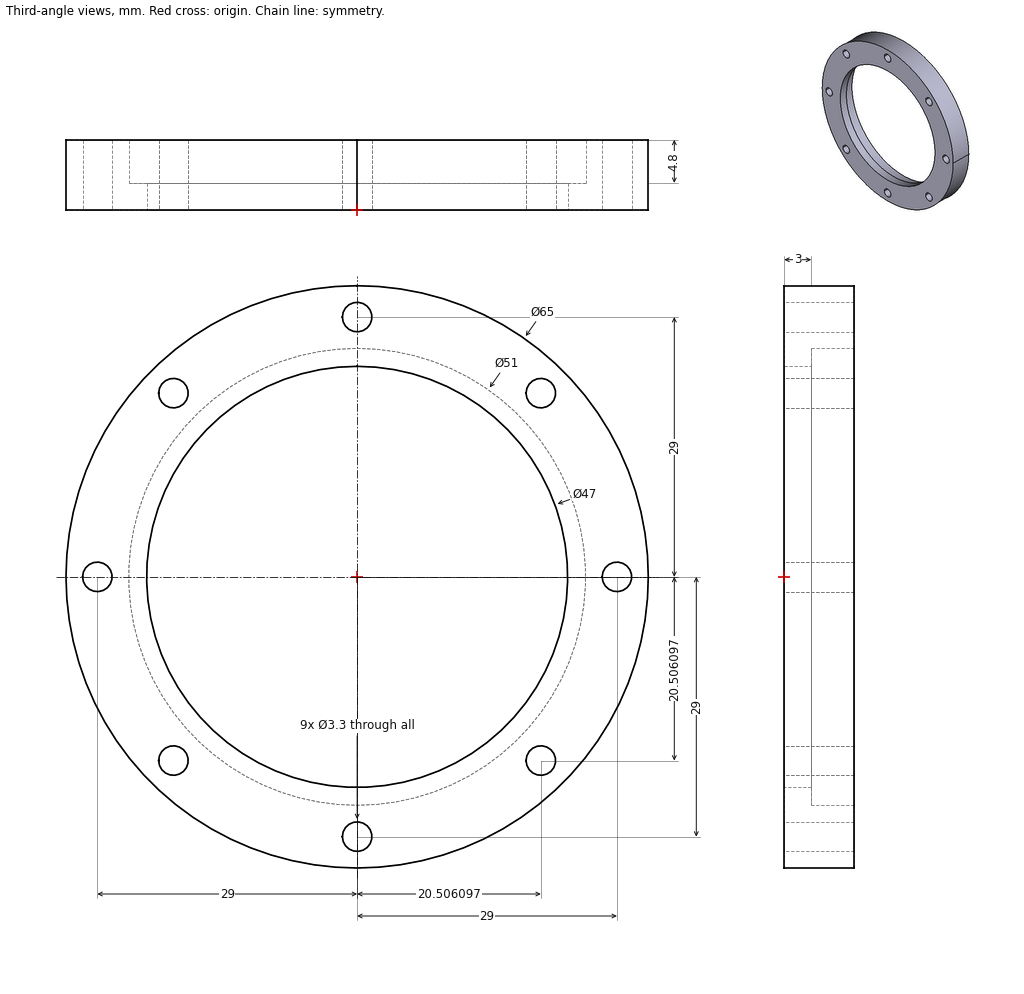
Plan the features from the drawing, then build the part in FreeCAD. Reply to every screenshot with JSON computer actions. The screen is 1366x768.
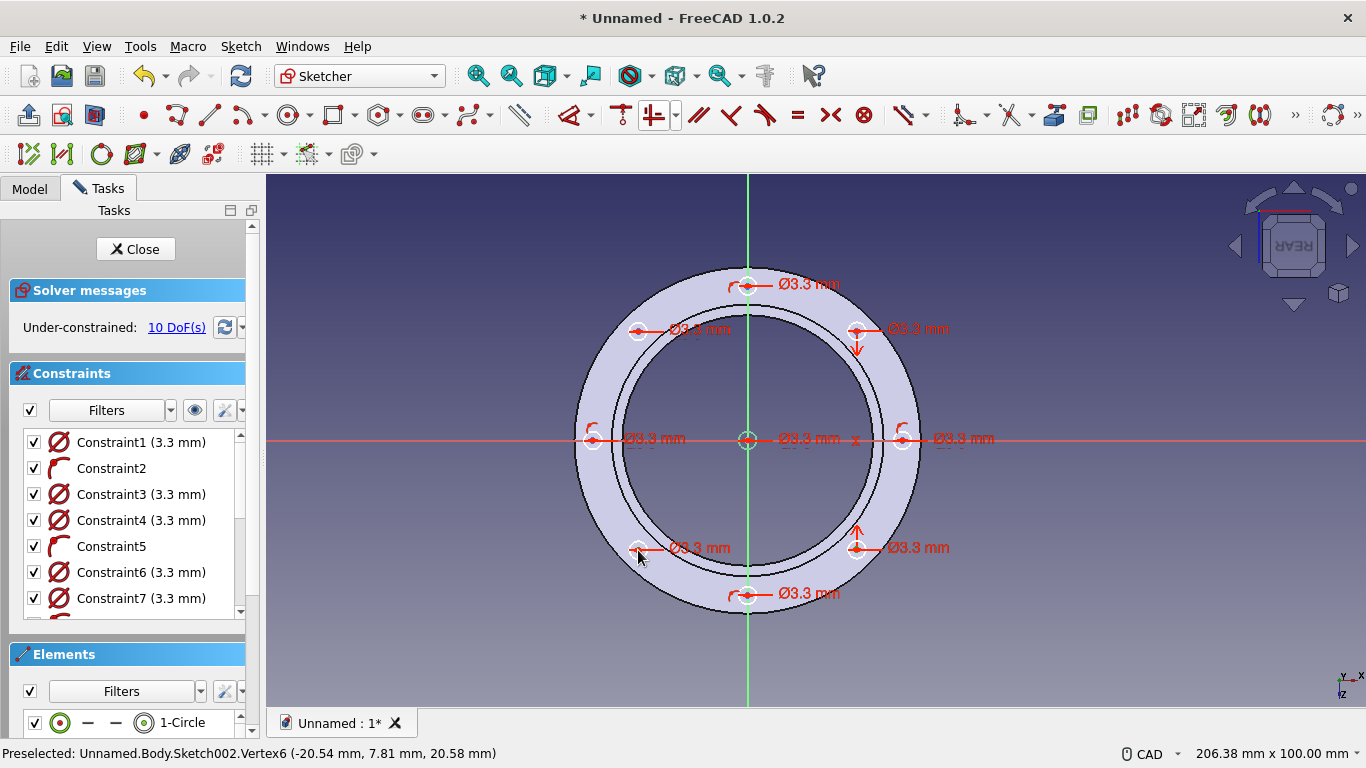
{"action": "left_click", "coordinate": [748, 645]}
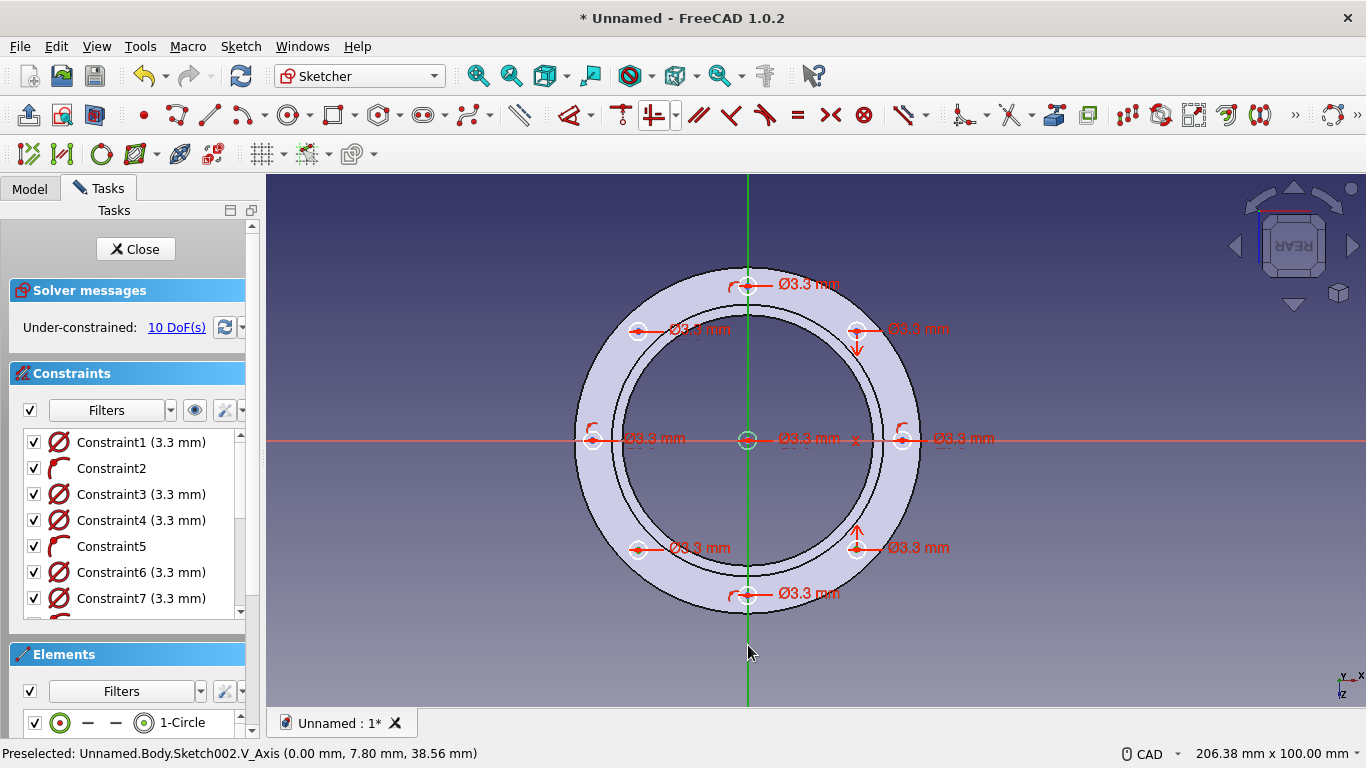
{"action": "left_click", "coordinate": [831, 116]}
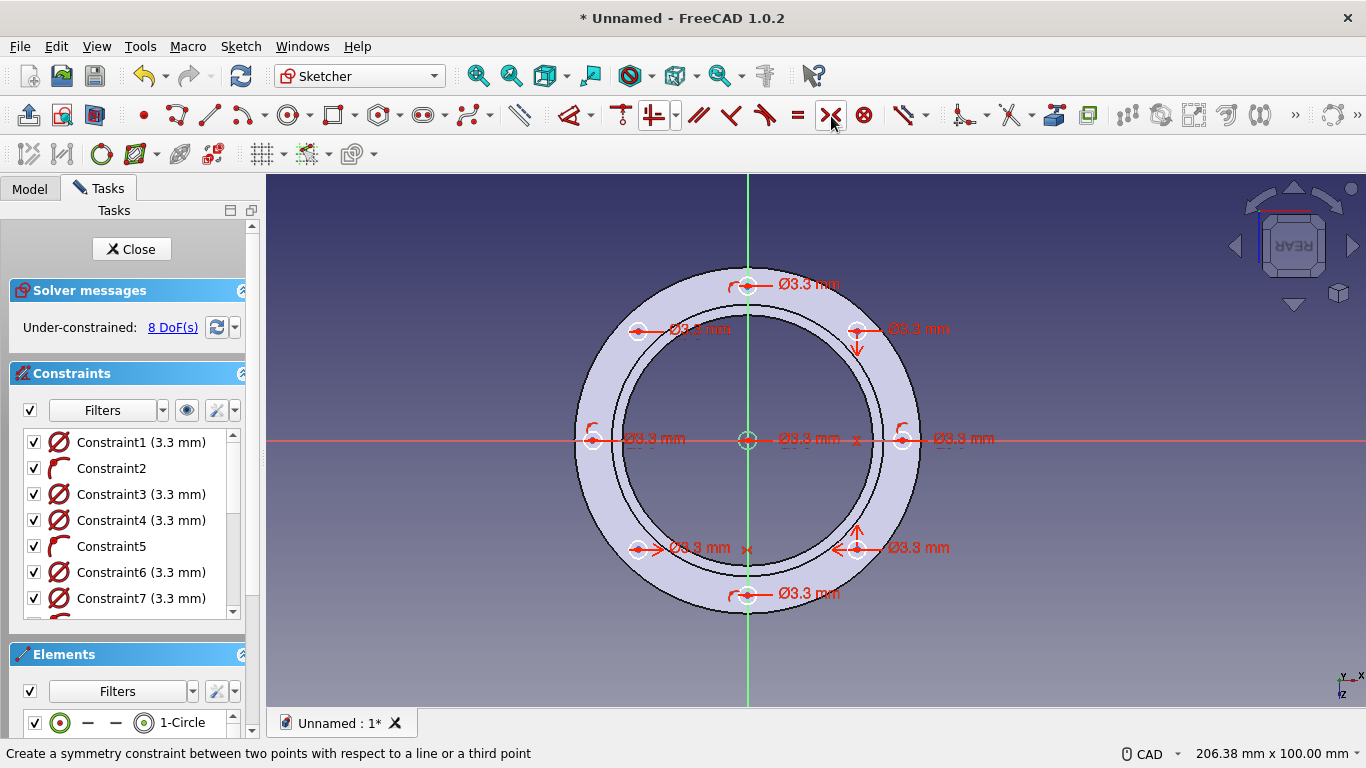
{"action": "left_click", "coordinate": [857, 331]}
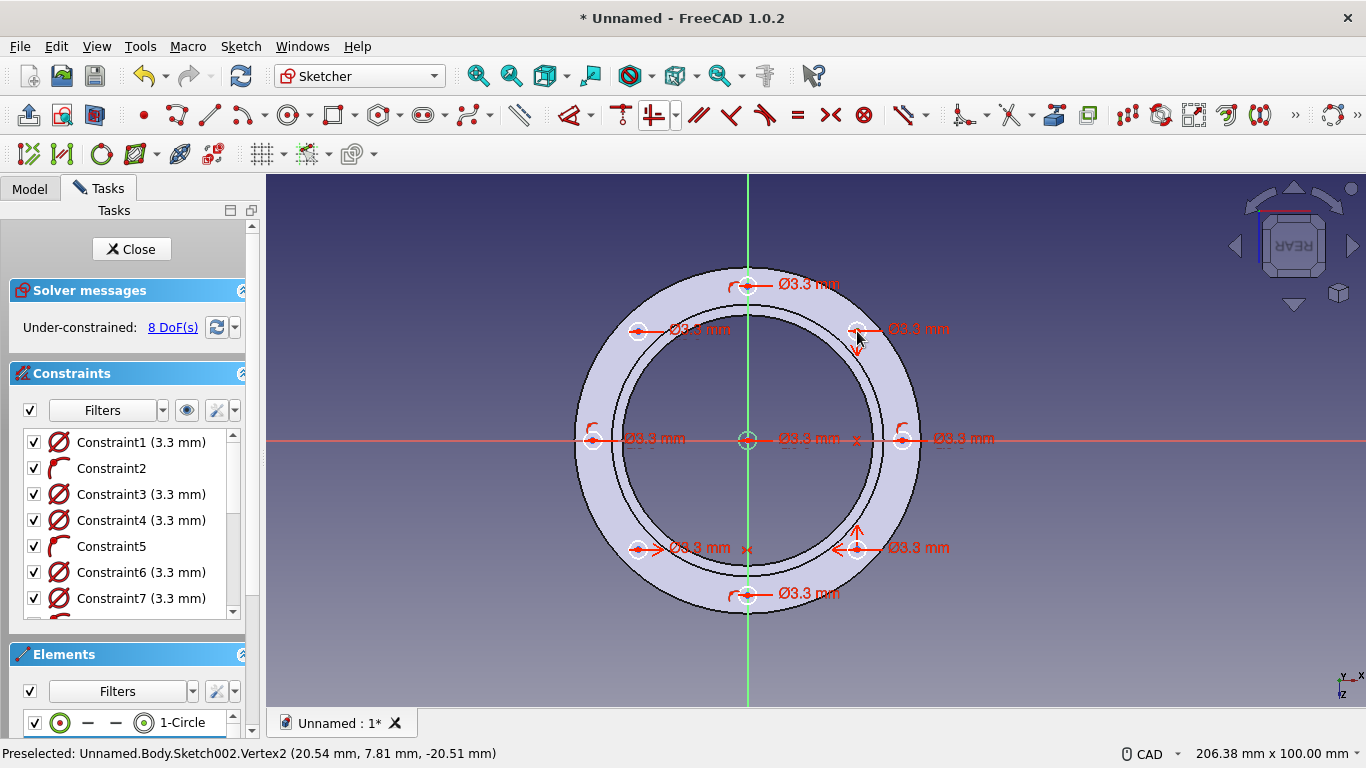
{"action": "left_click", "coordinate": [638, 332]}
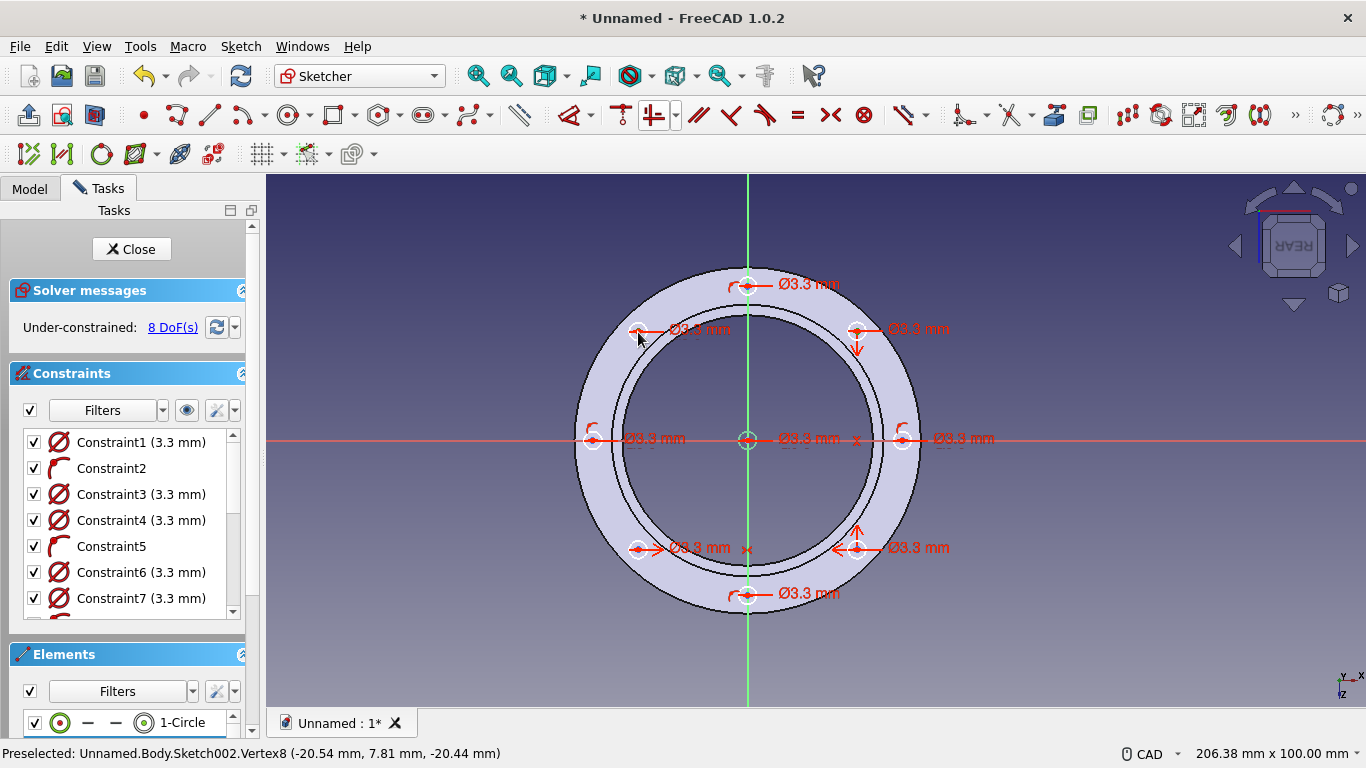
{"action": "left_click", "coordinate": [748, 645]}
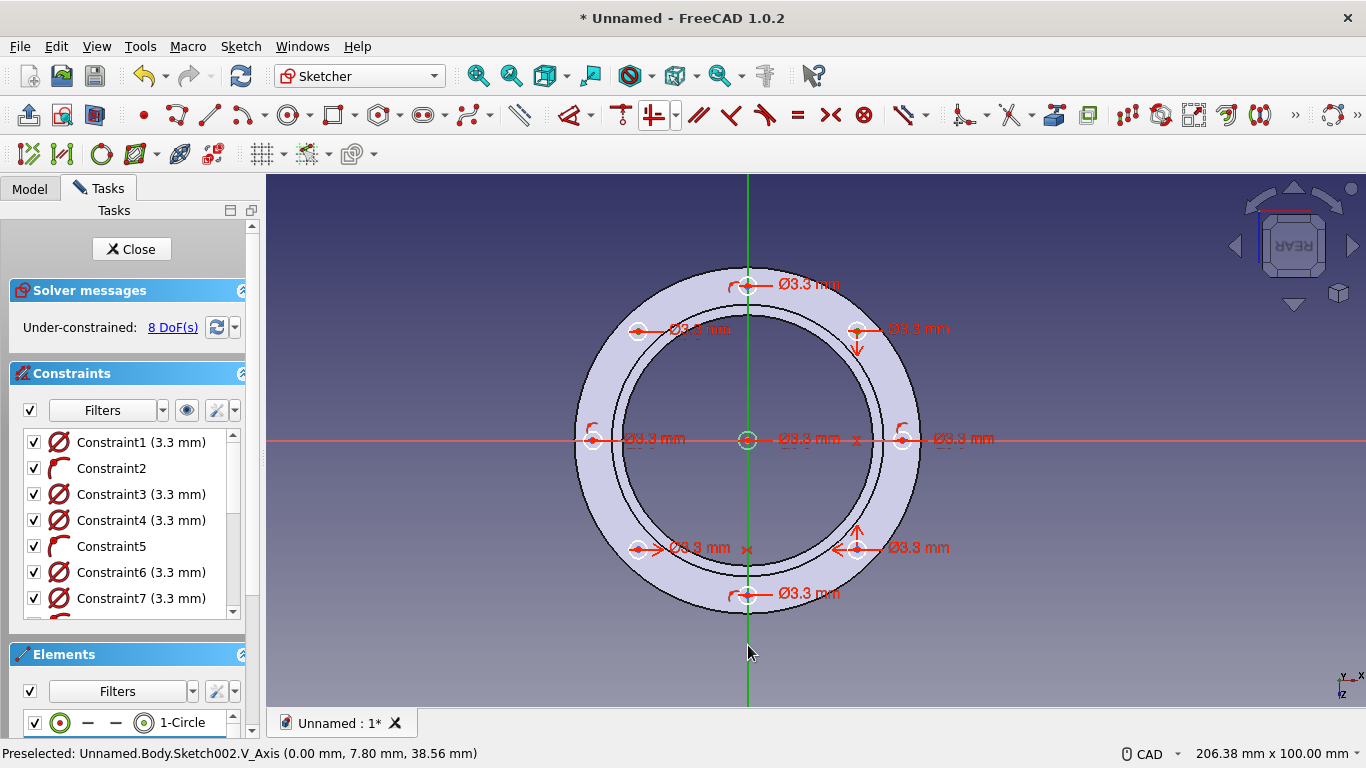
{"action": "left_click", "coordinate": [831, 116]}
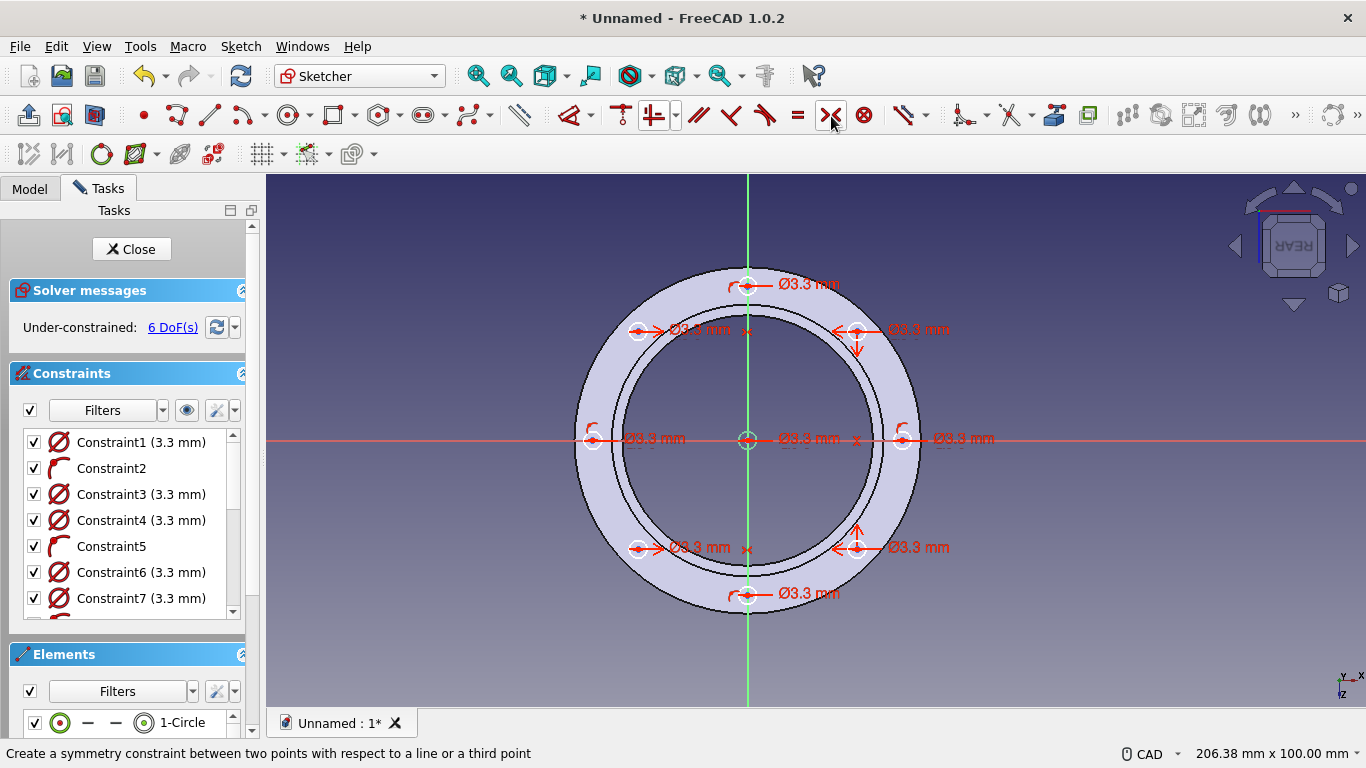
{"action": "left_click", "coordinate": [568, 116]}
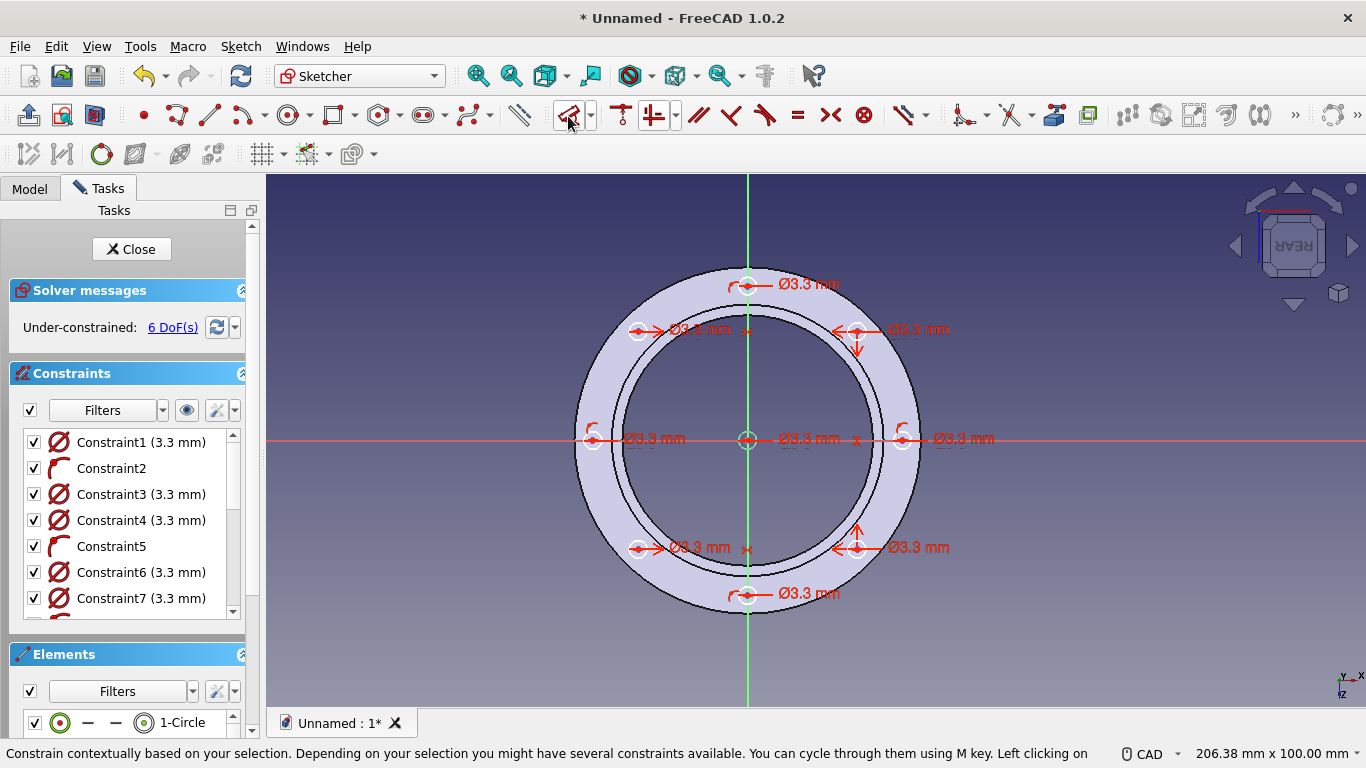
{"action": "left_click", "coordinate": [748, 286]}
{"action": "left_click", "coordinate": [782, 363]}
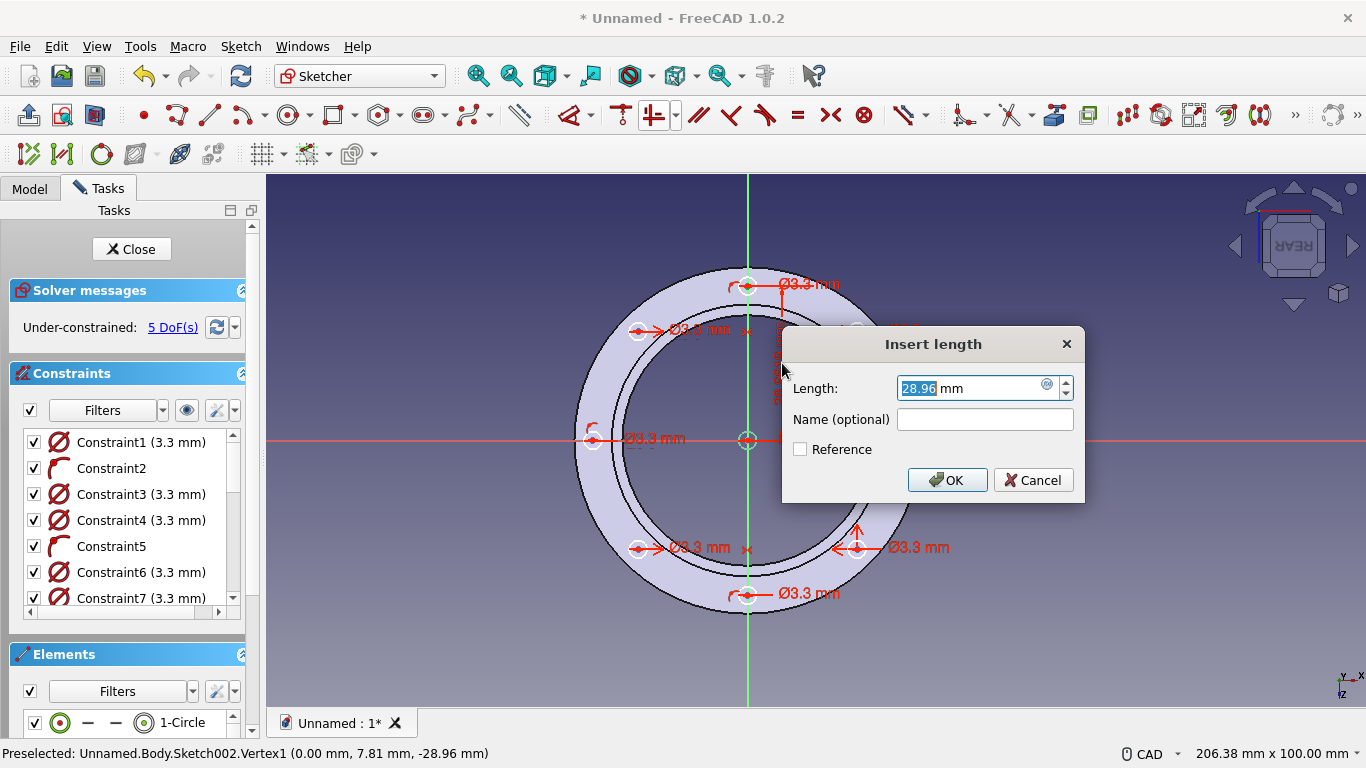
{"action": "type", "text": "29"}
{"action": "key", "text": "Return"}